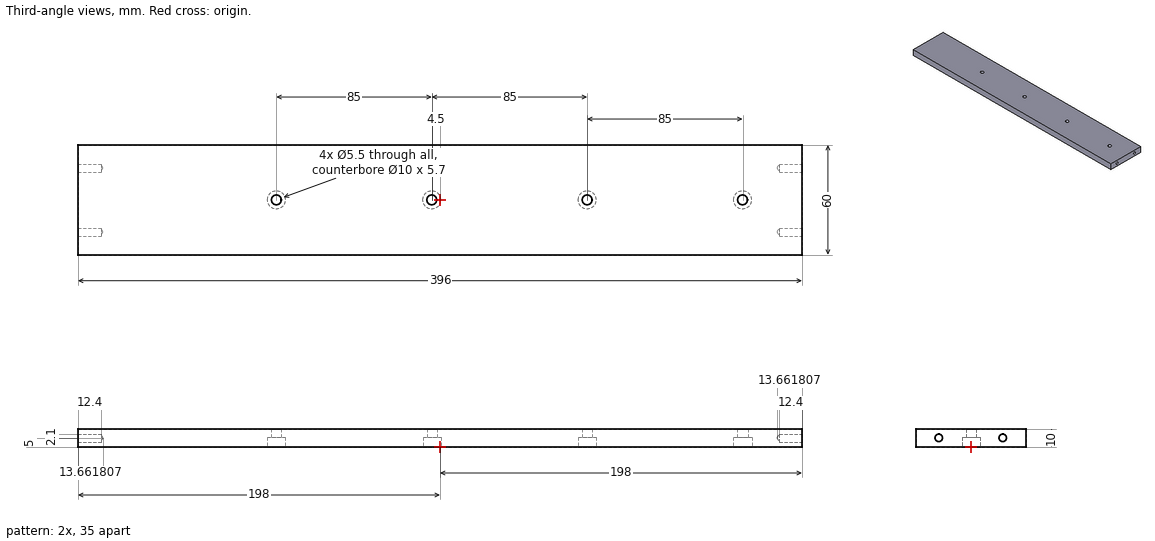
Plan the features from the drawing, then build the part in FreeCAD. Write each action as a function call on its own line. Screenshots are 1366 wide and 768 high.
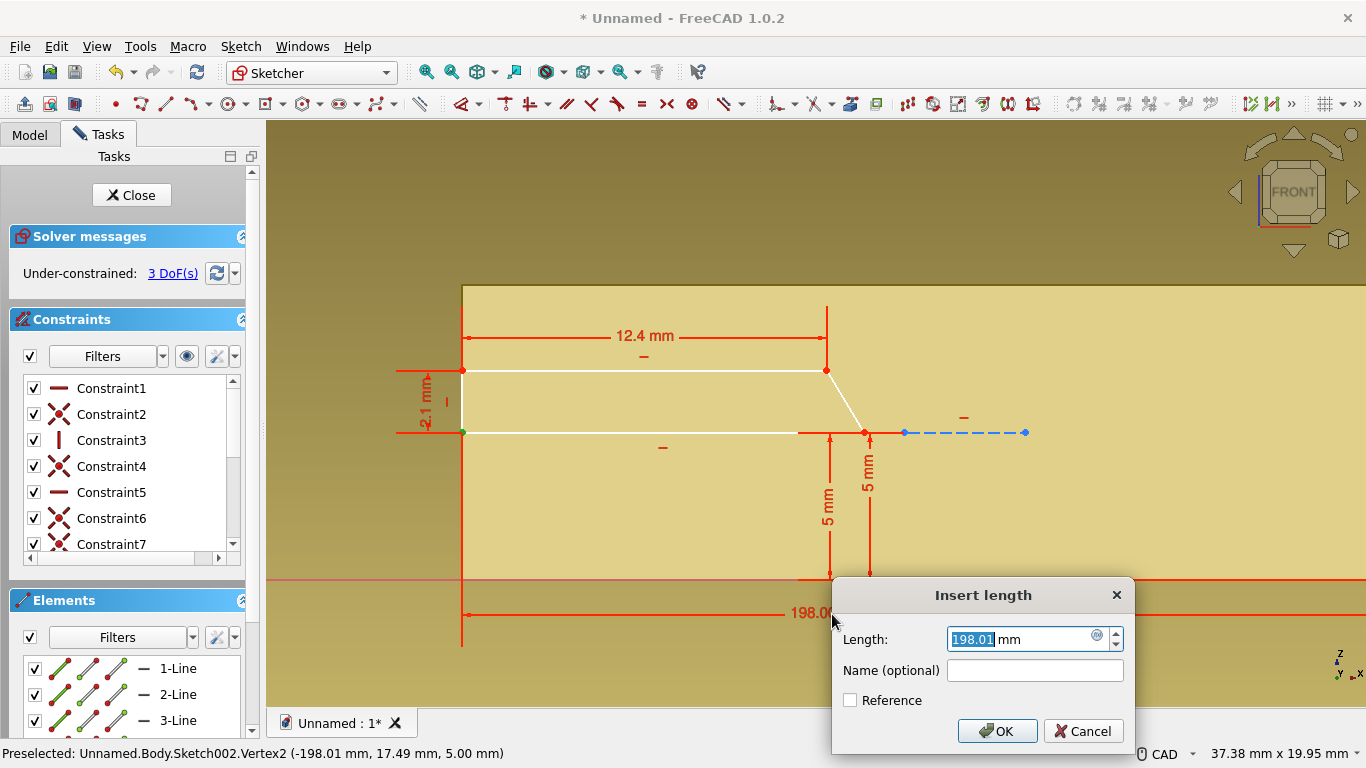
text(198)
key(Return)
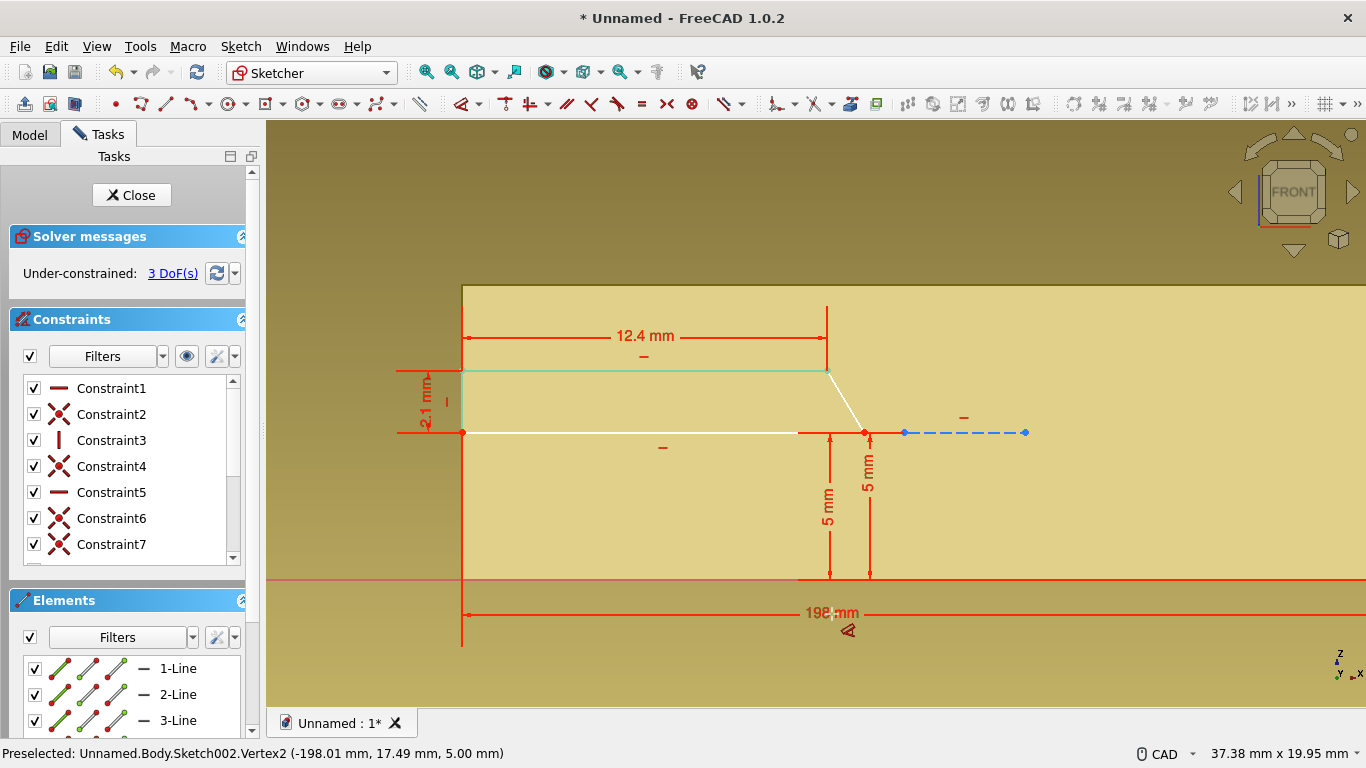
click(743, 433)
click(663, 467)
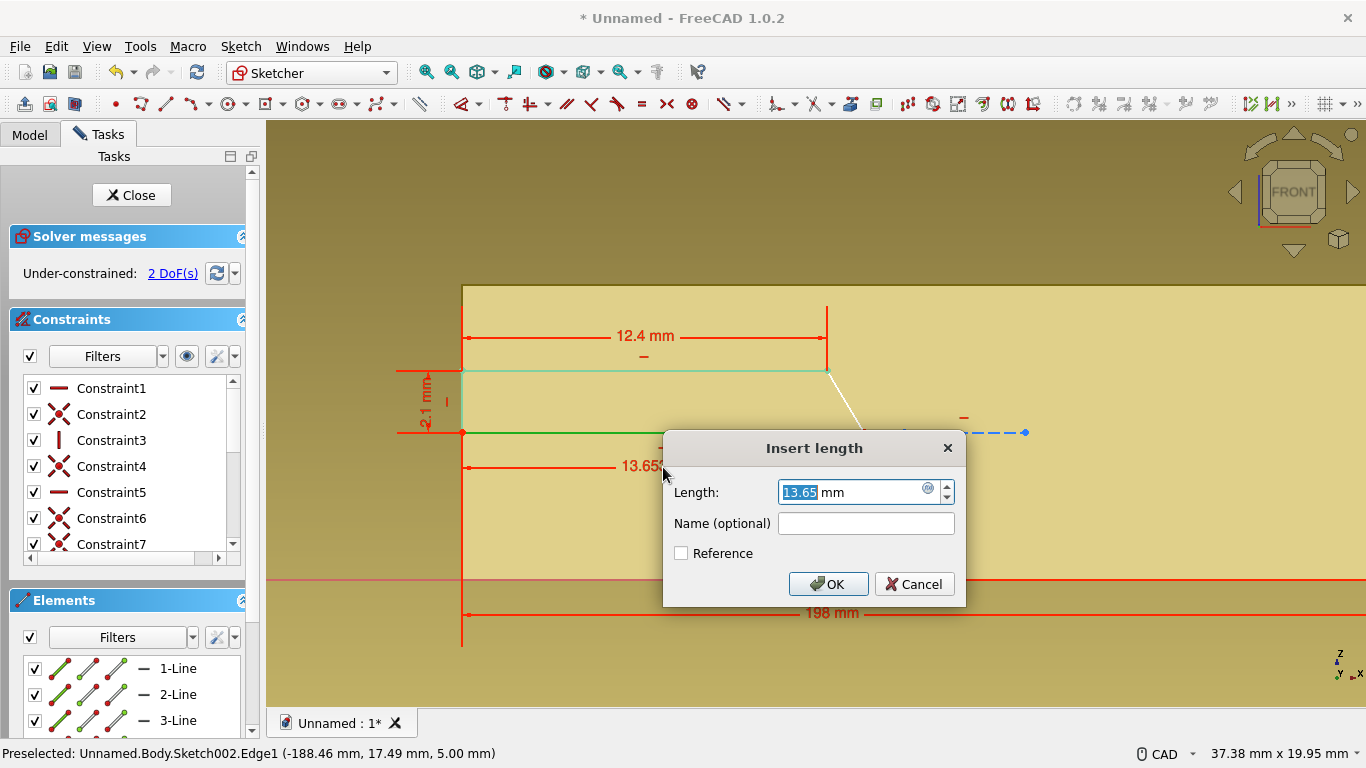
text(13.661807)
key(Return)
key(Escape)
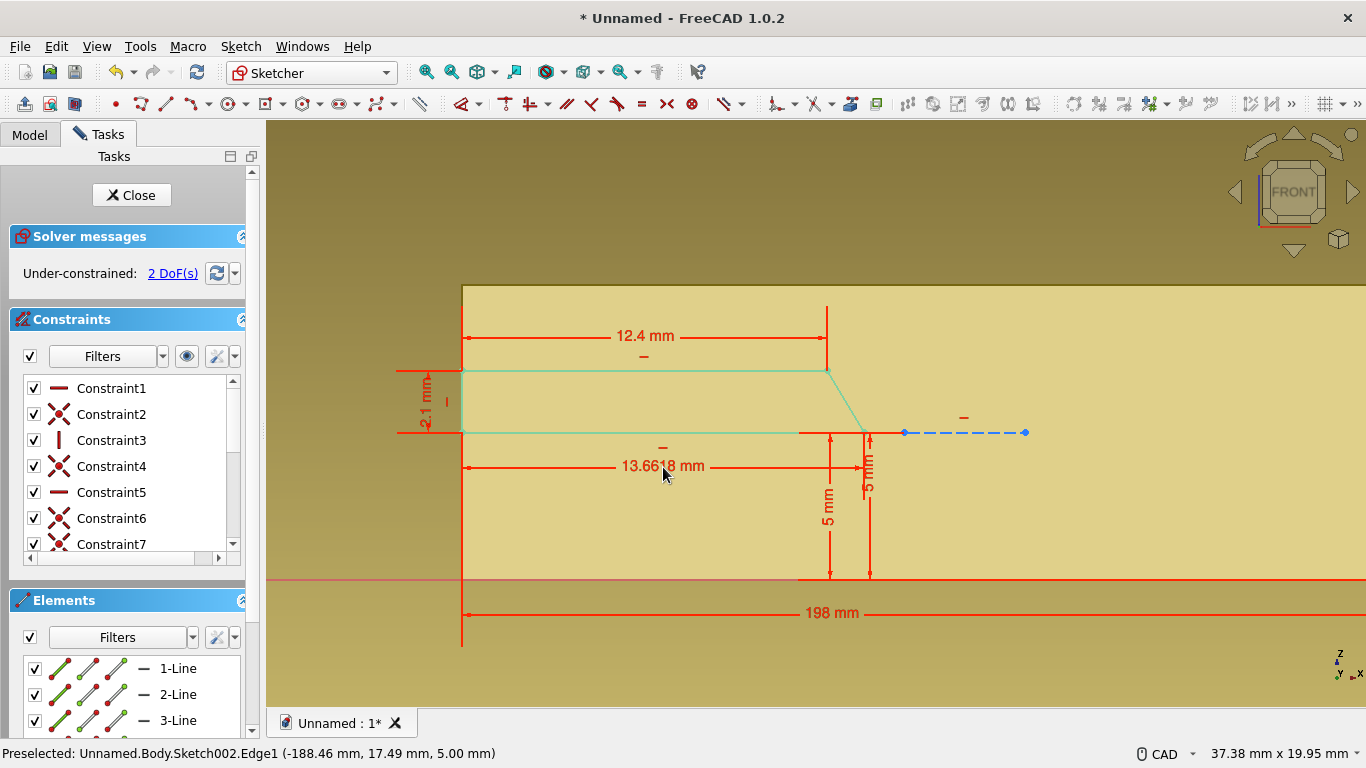
click(132, 195)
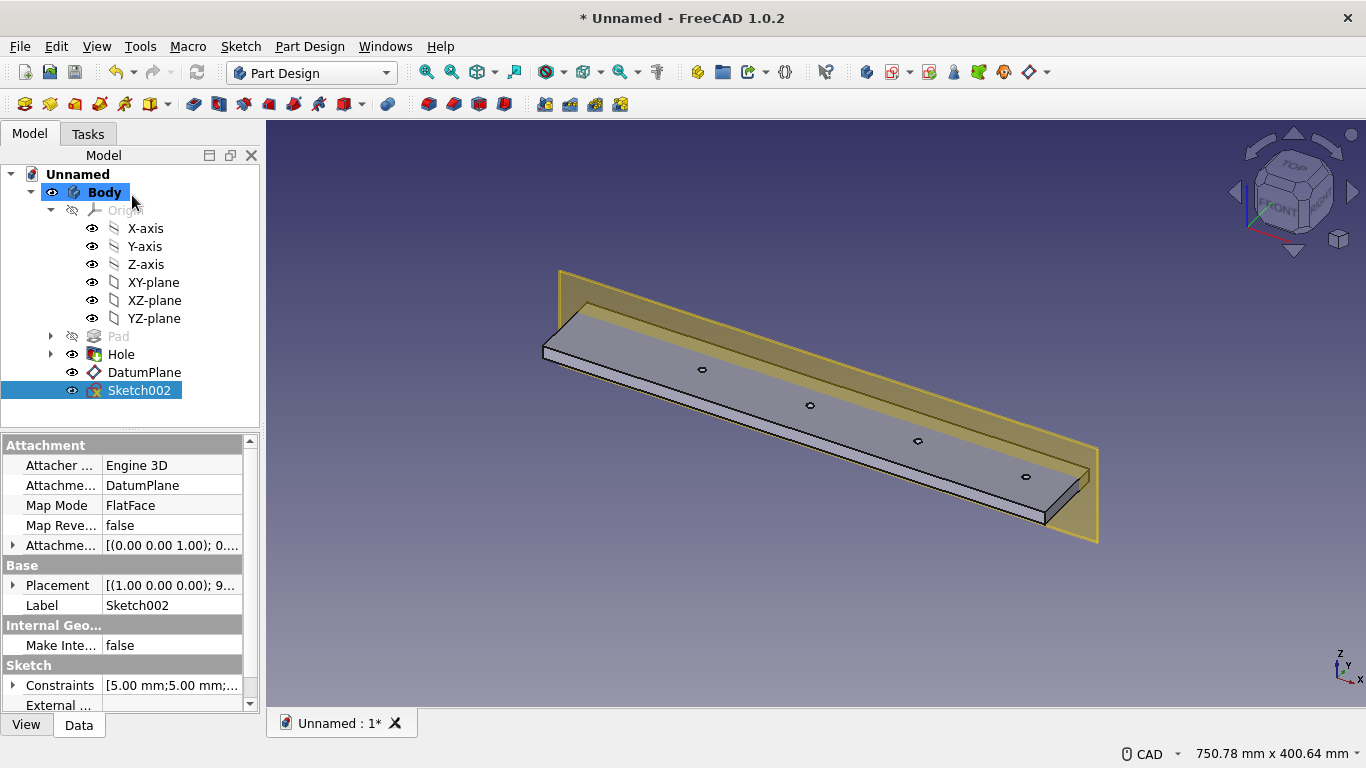
click(244, 104)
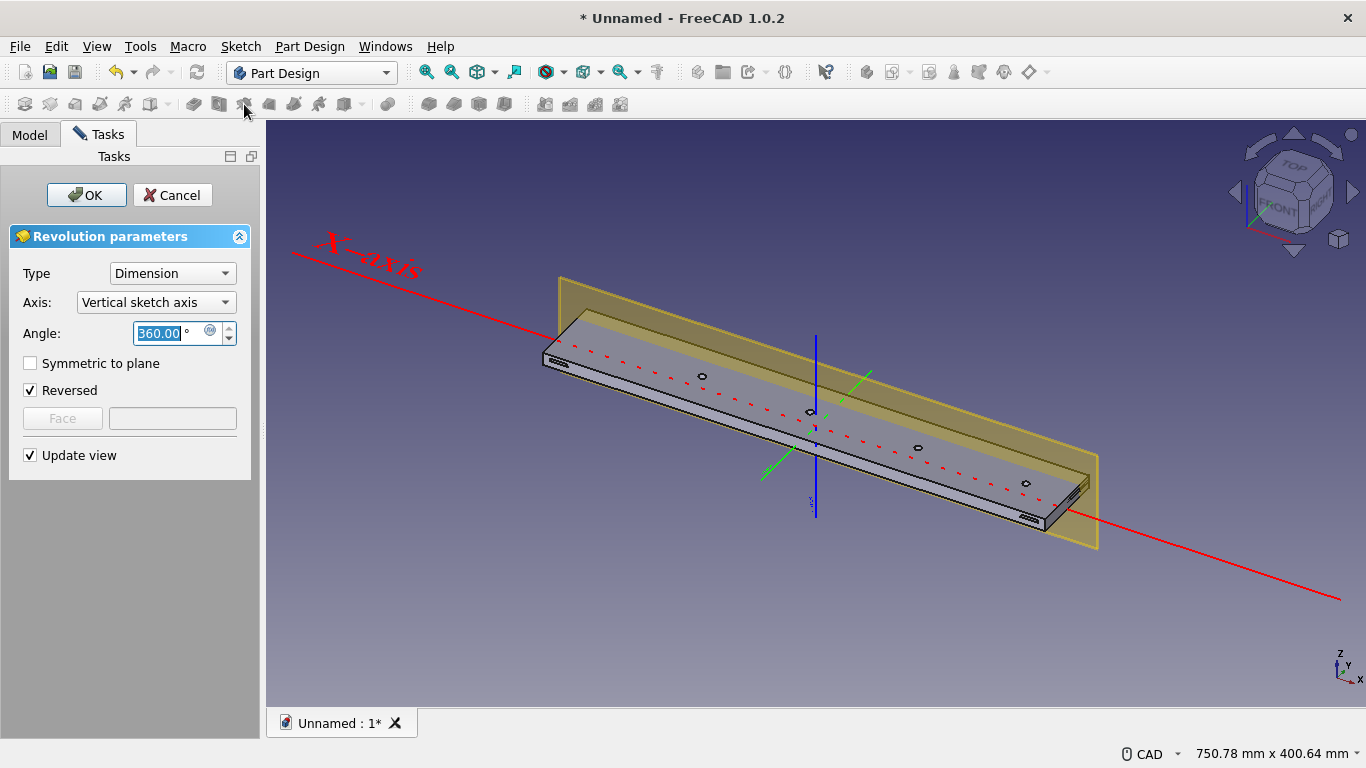
click(157, 302)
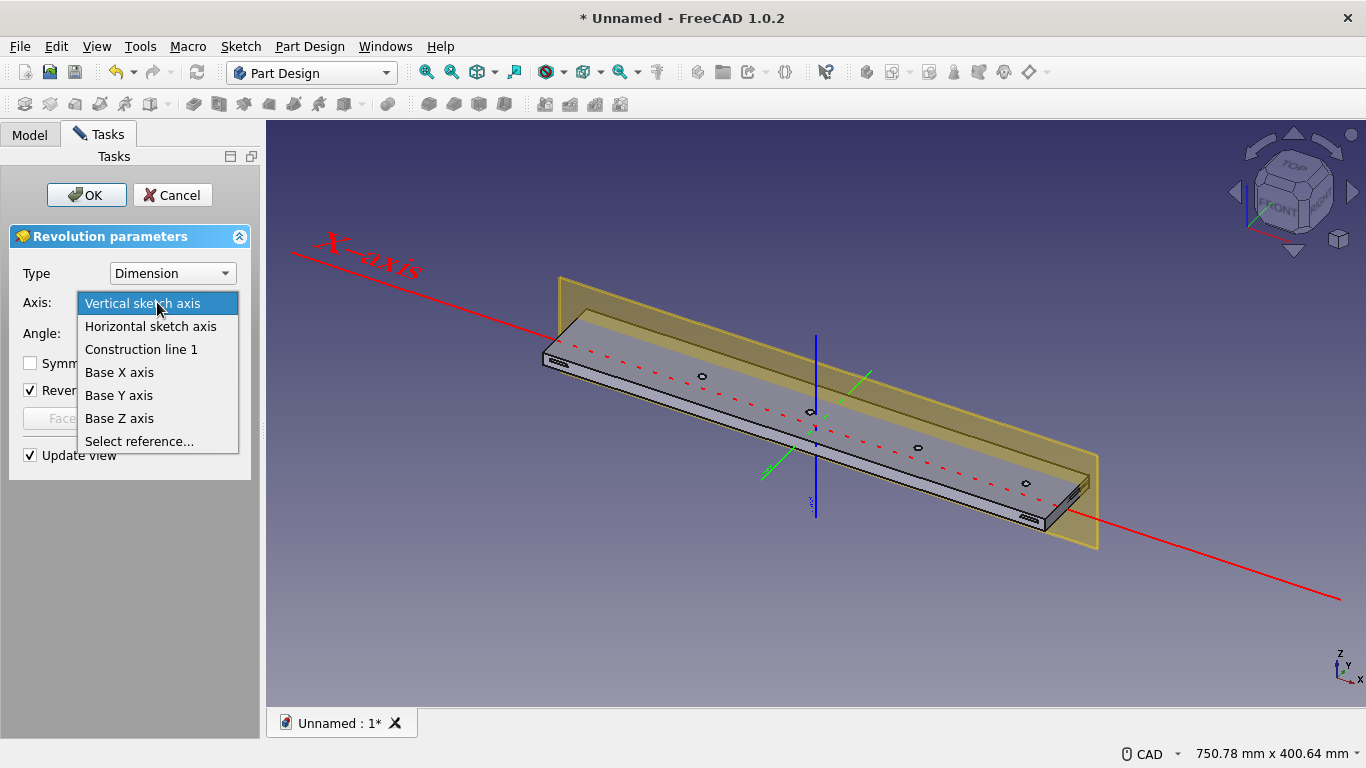
click(156, 350)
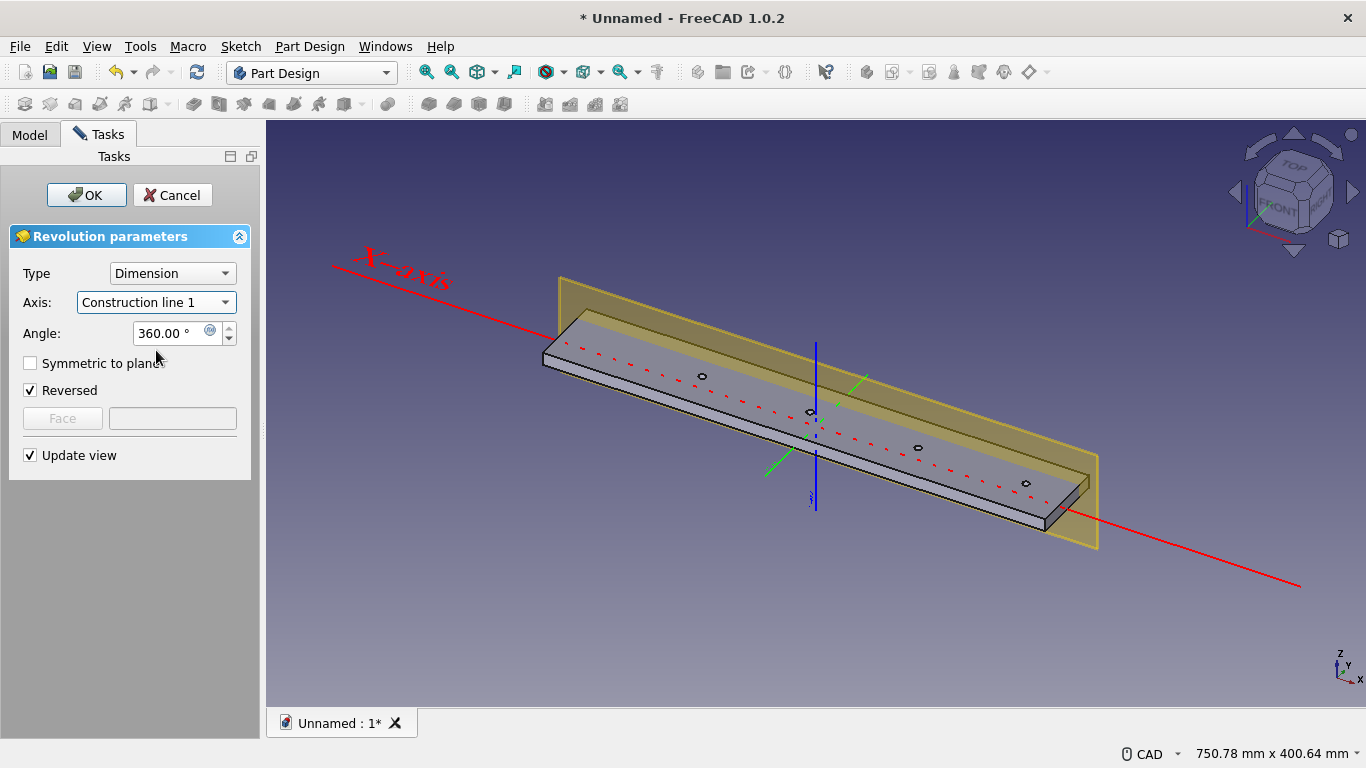
click(87, 195)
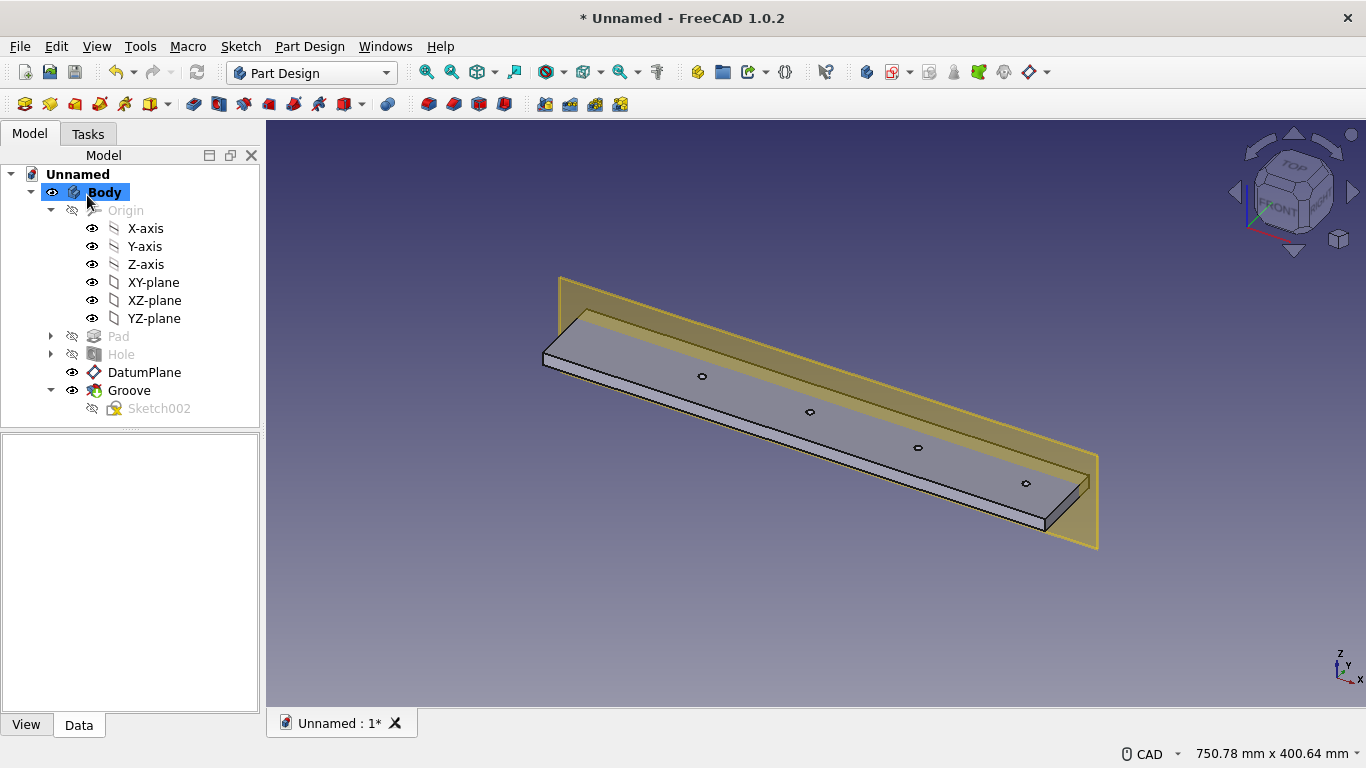
click(117, 372)
key(space)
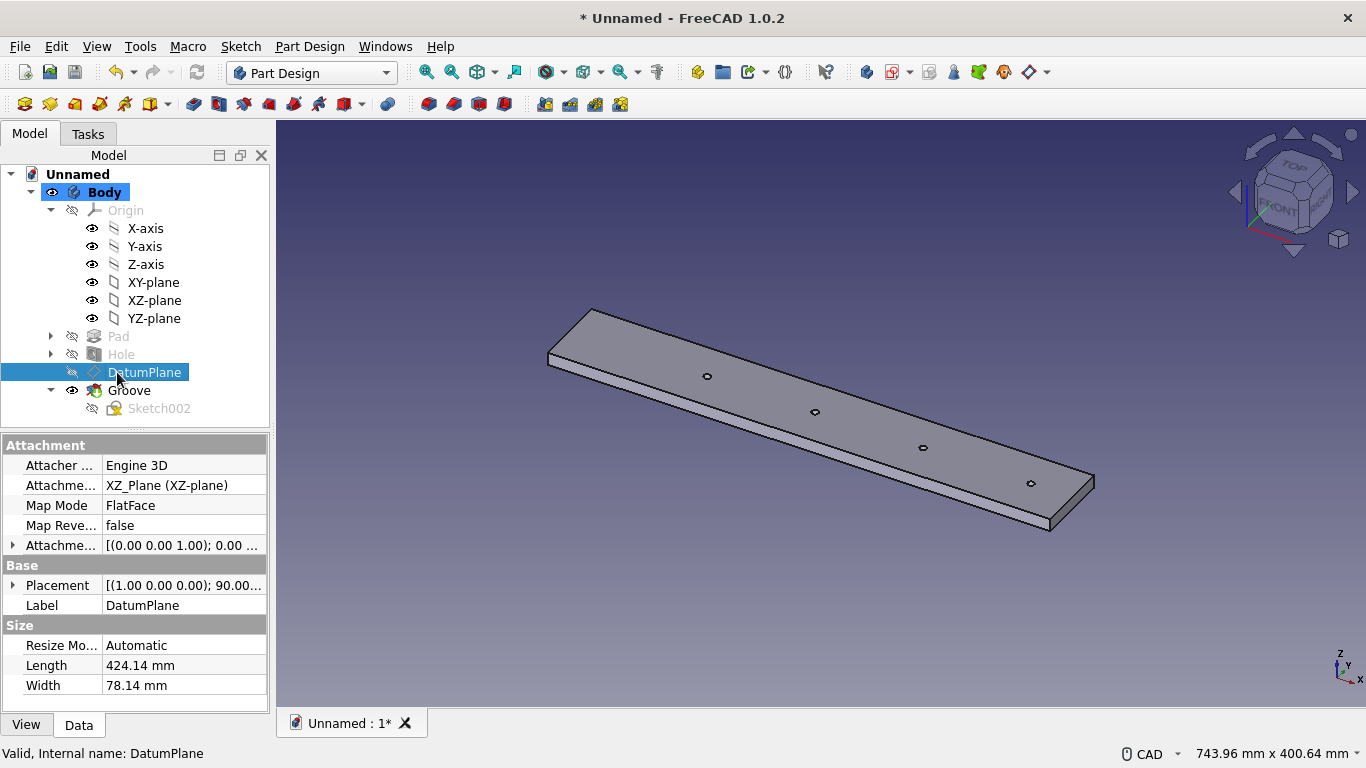
click(117, 390)